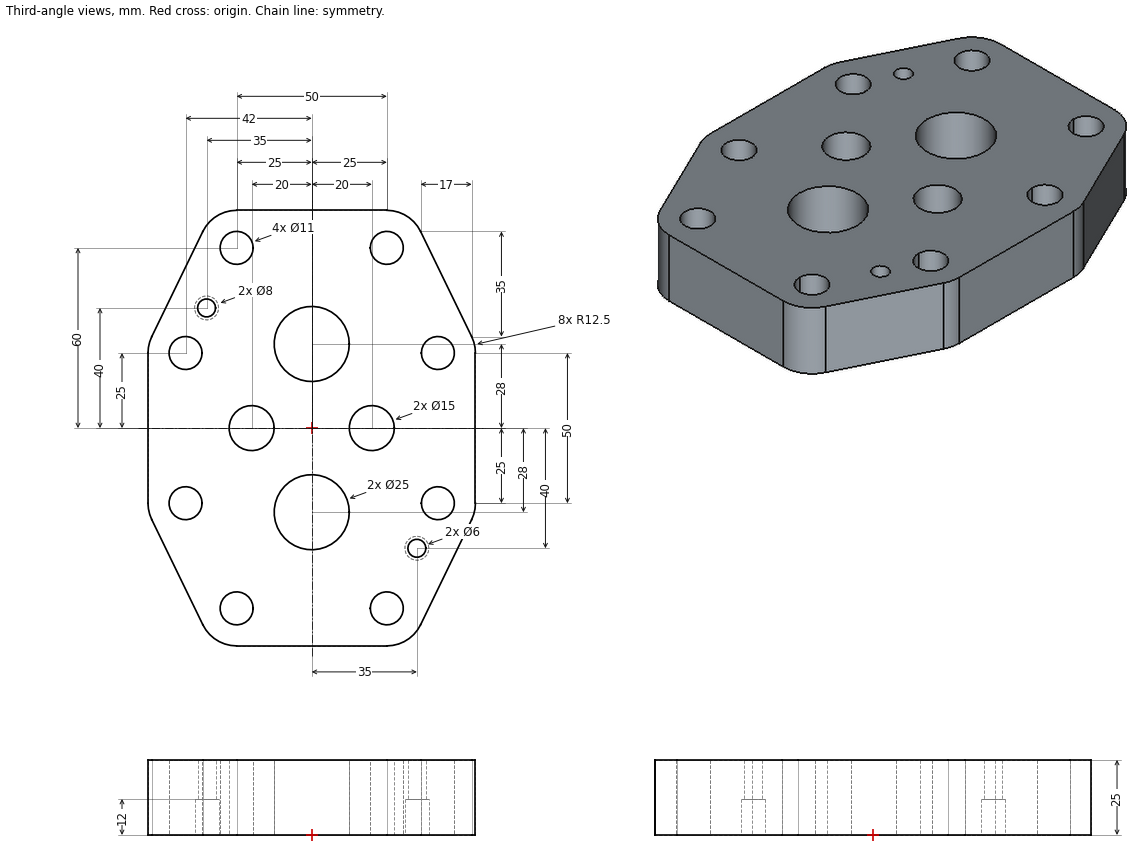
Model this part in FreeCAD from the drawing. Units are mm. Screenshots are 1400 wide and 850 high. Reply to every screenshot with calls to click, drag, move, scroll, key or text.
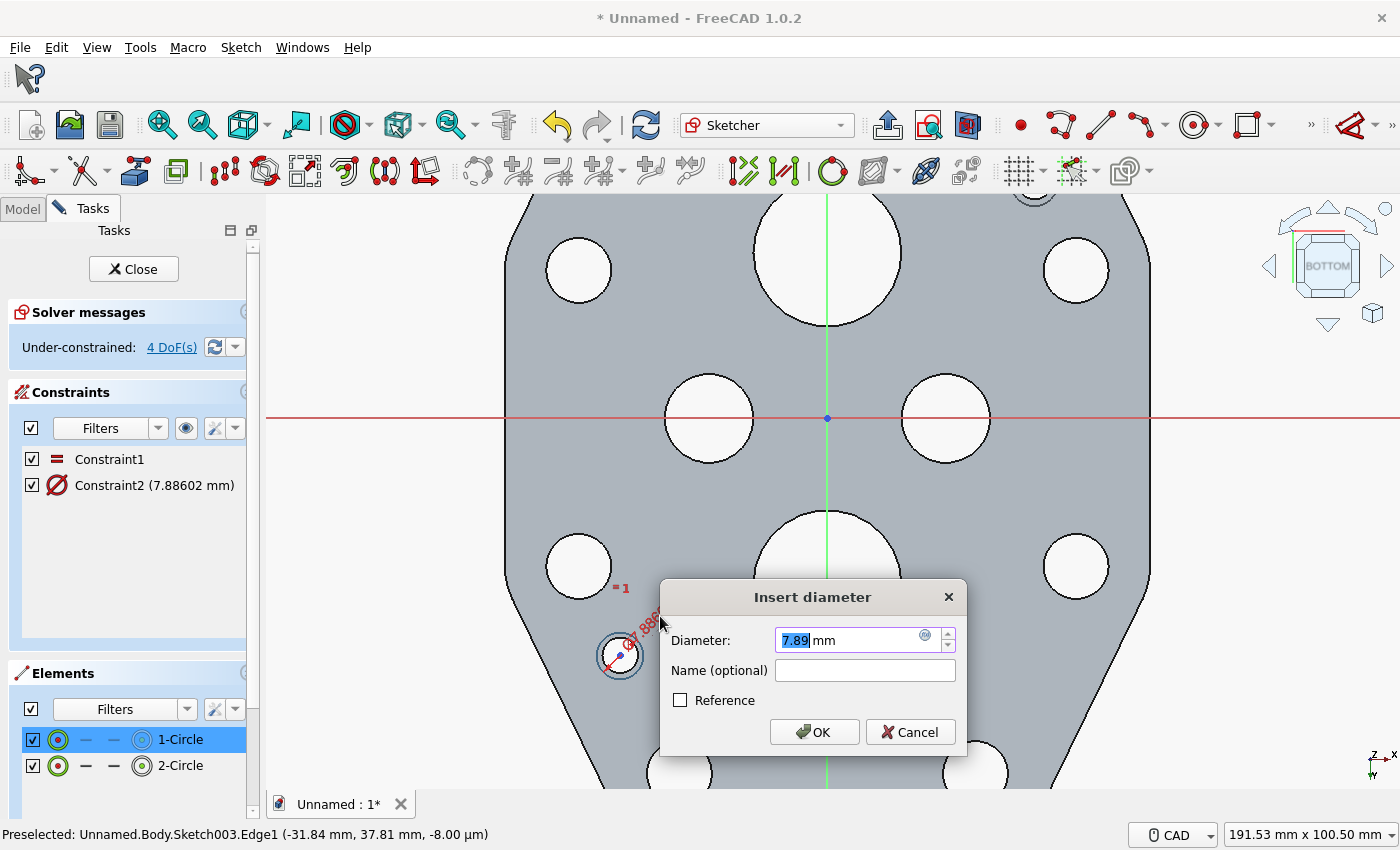
text(8)
key(Return)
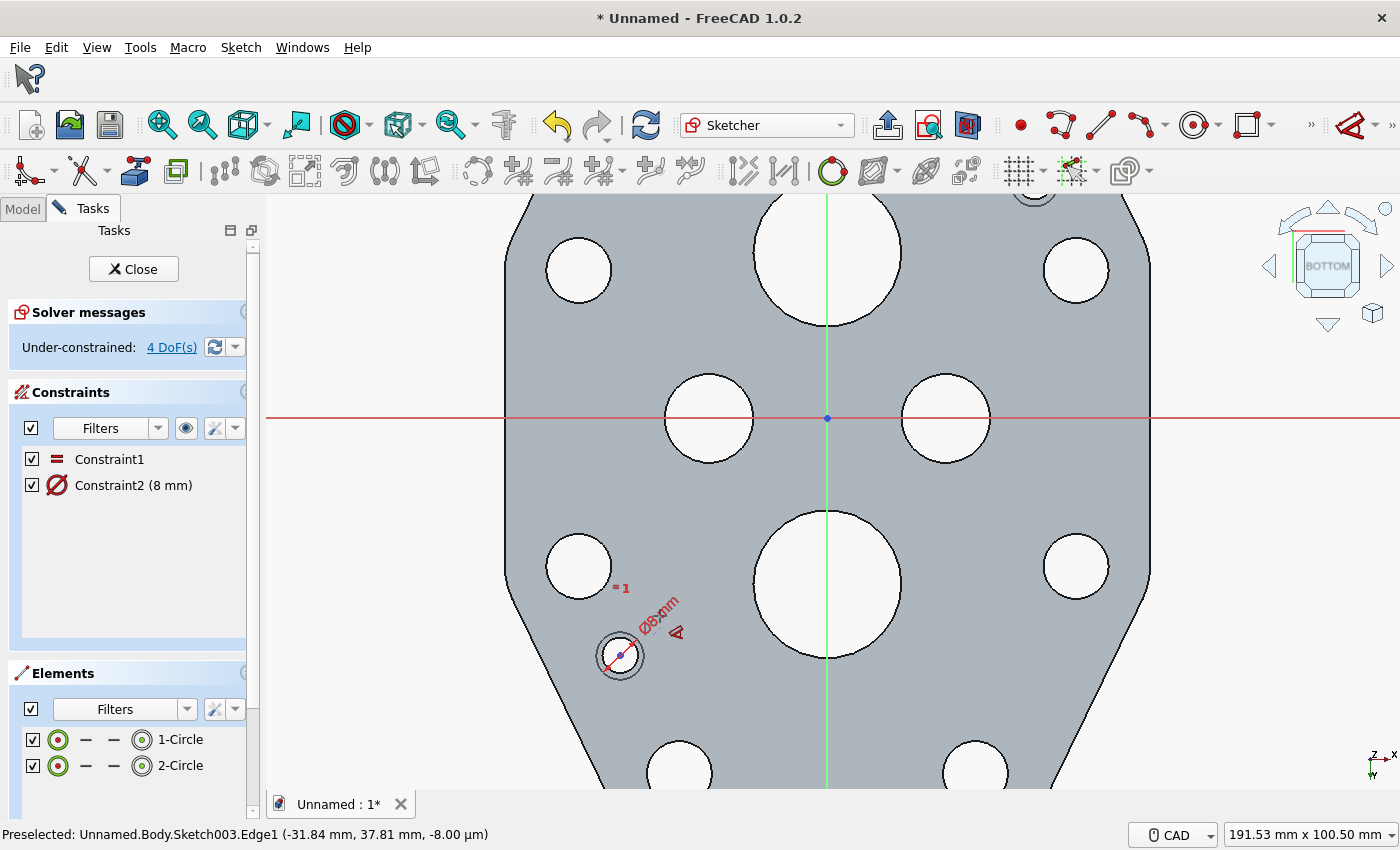
click(620, 656)
click(724, 690)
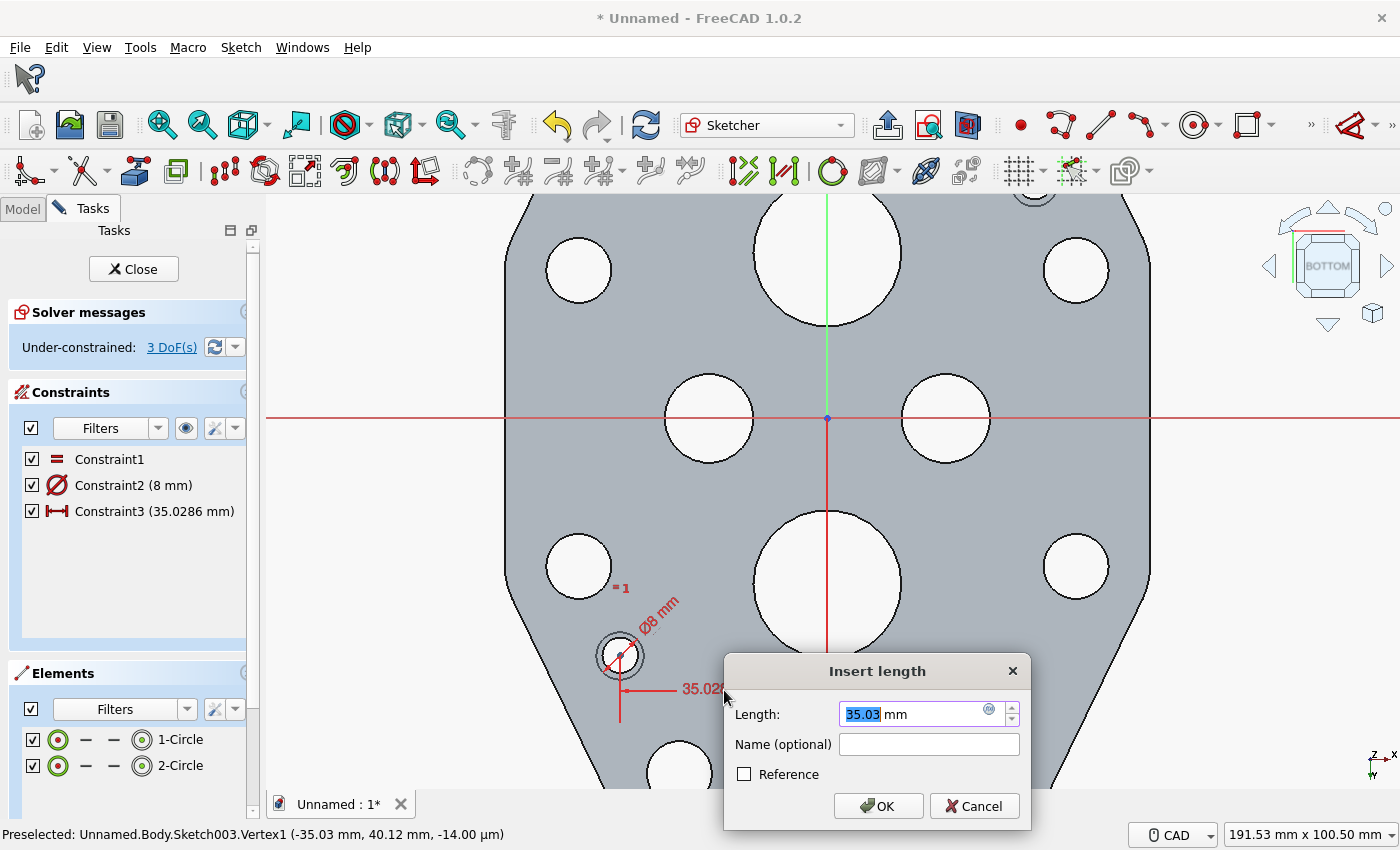
text(35)
key(Return)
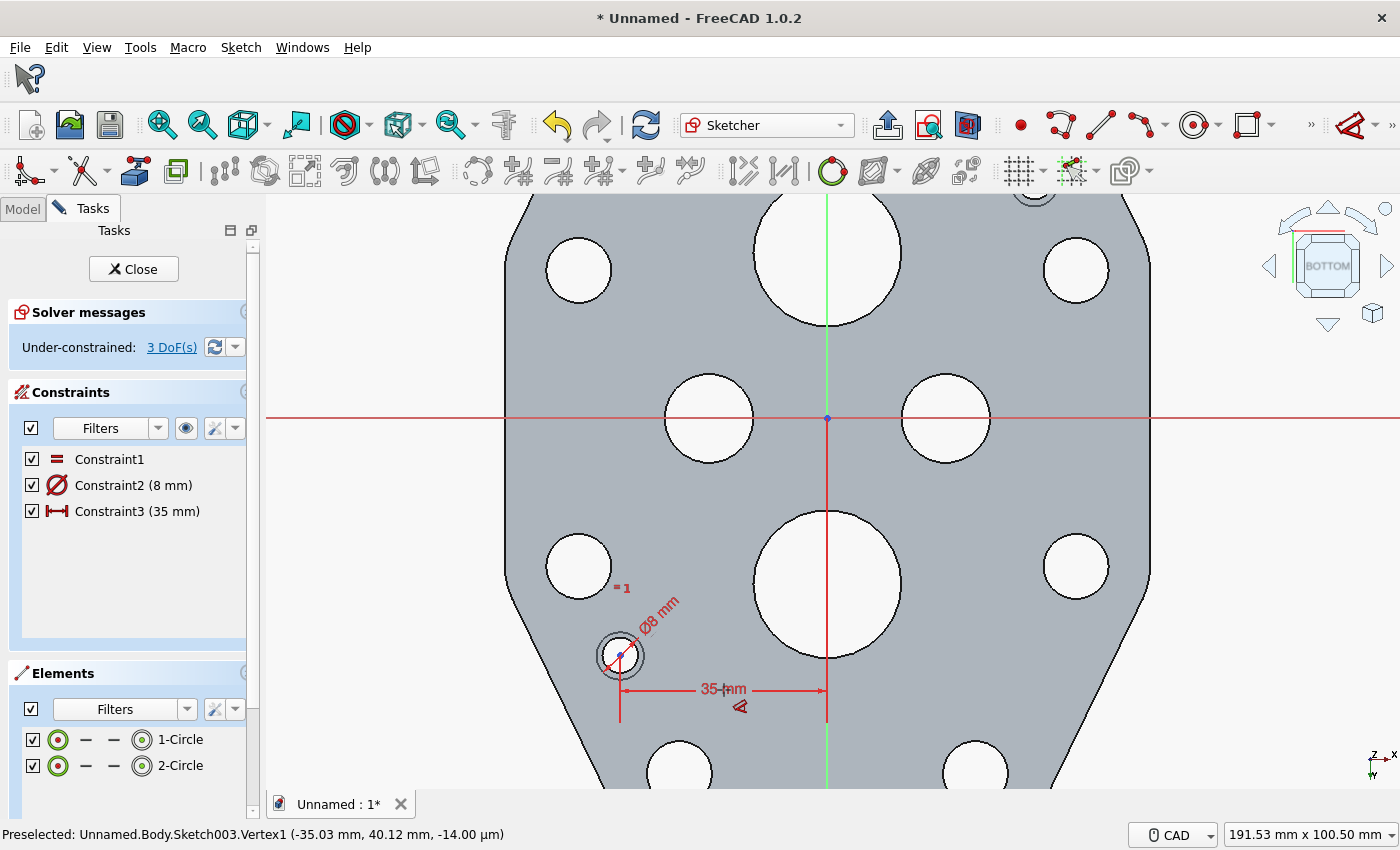
click(620, 656)
click(586, 537)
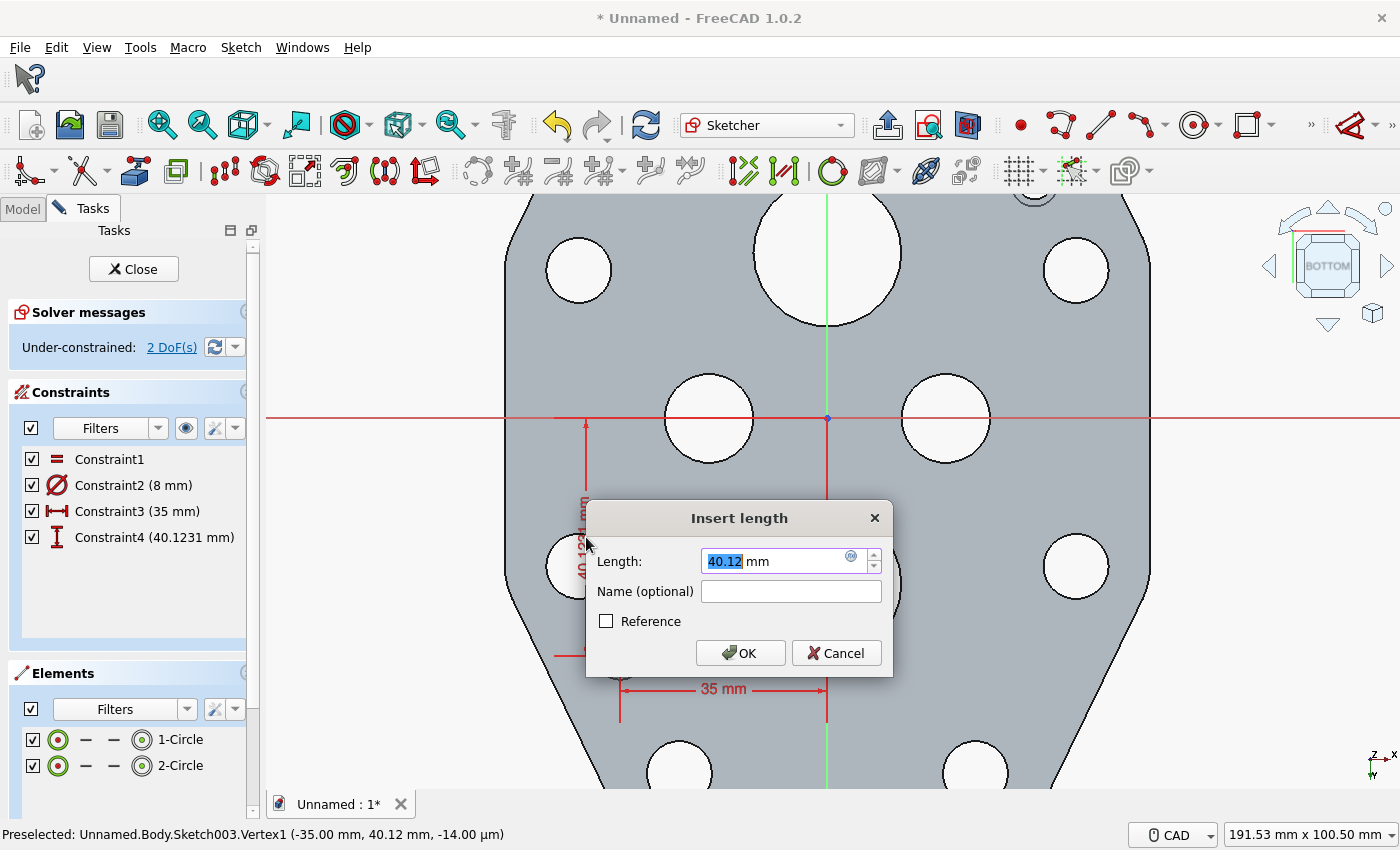
text(40)
key(Return)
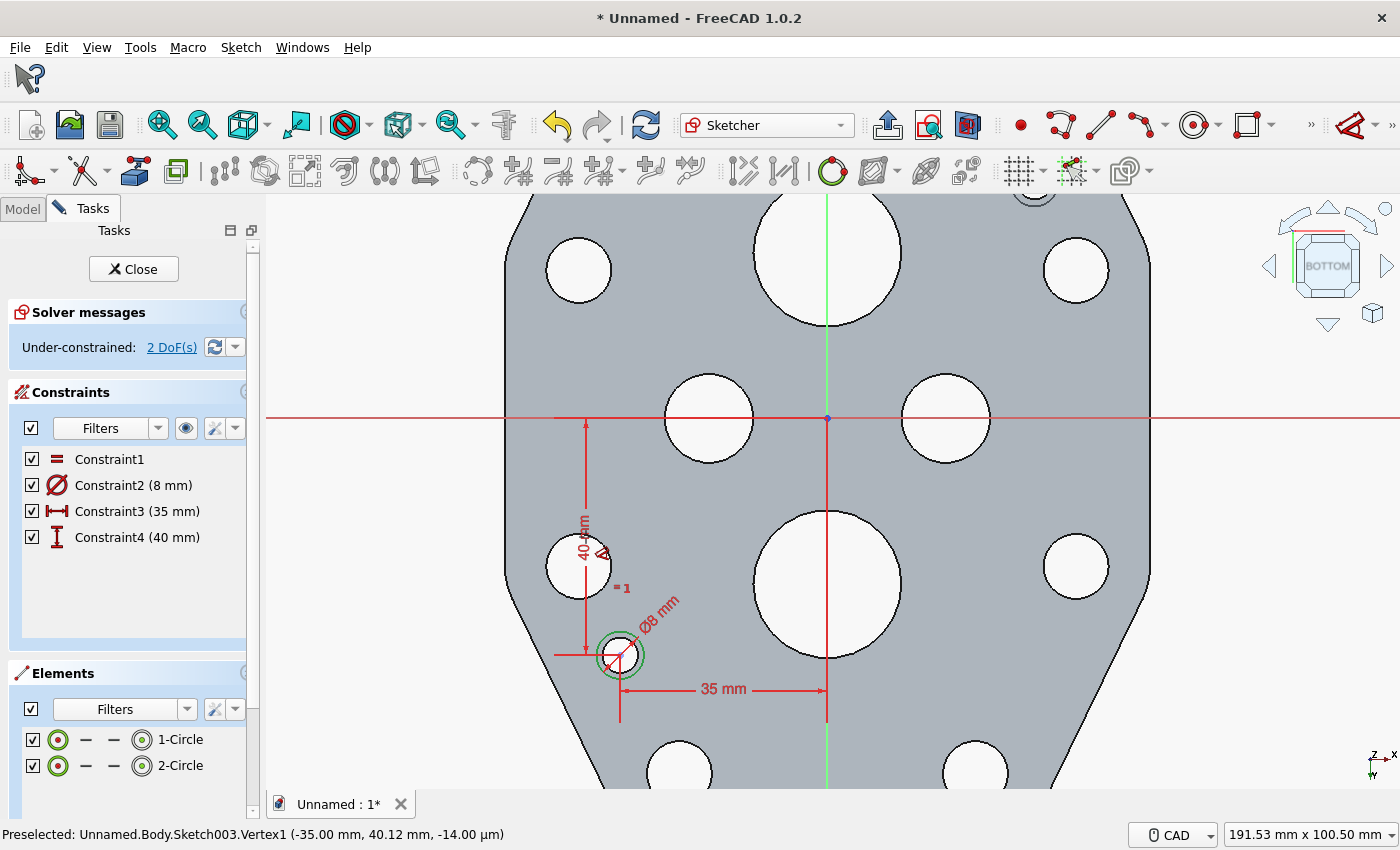
scroll(637, 640, down, 2)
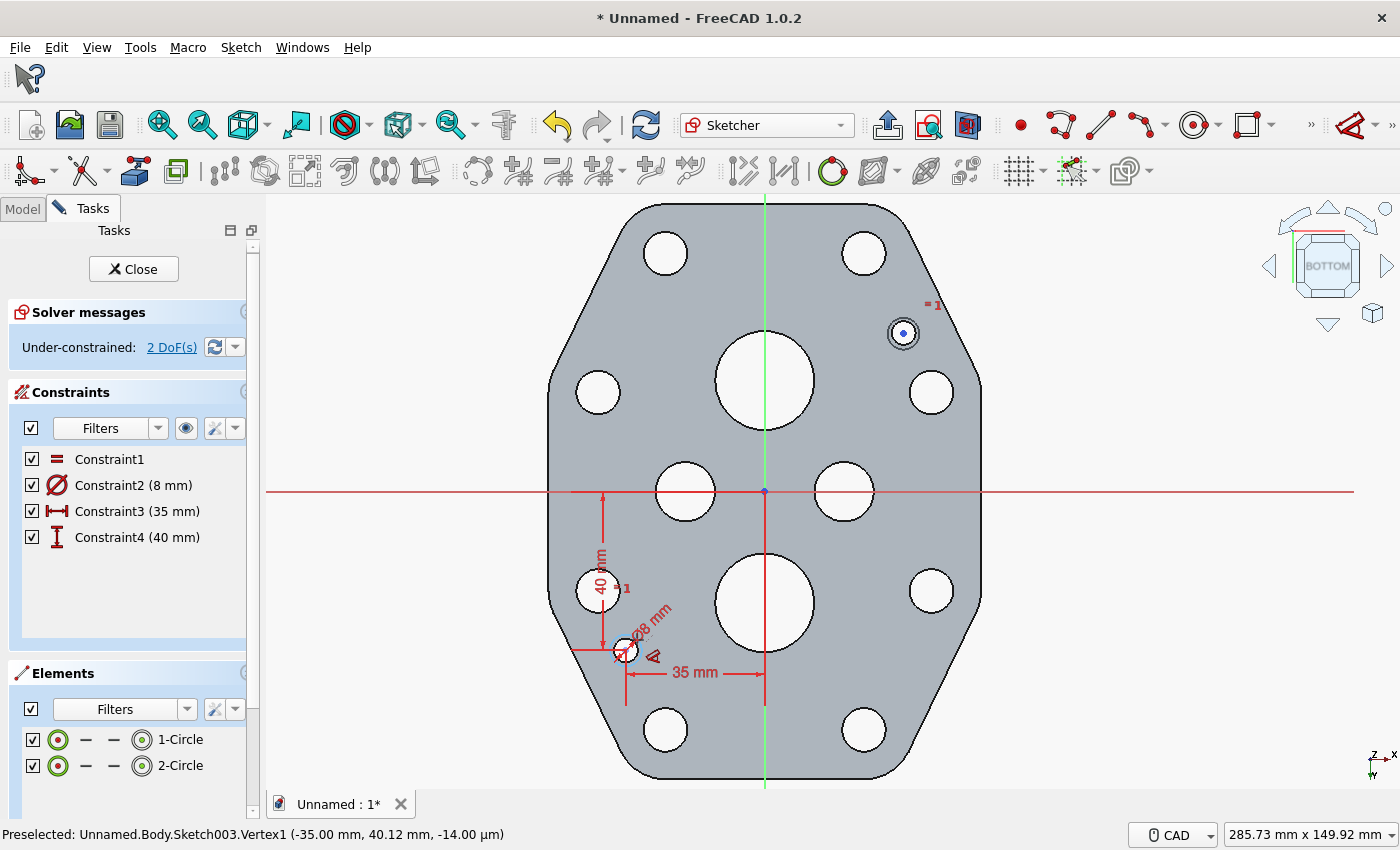
click(904, 334)
click(834, 300)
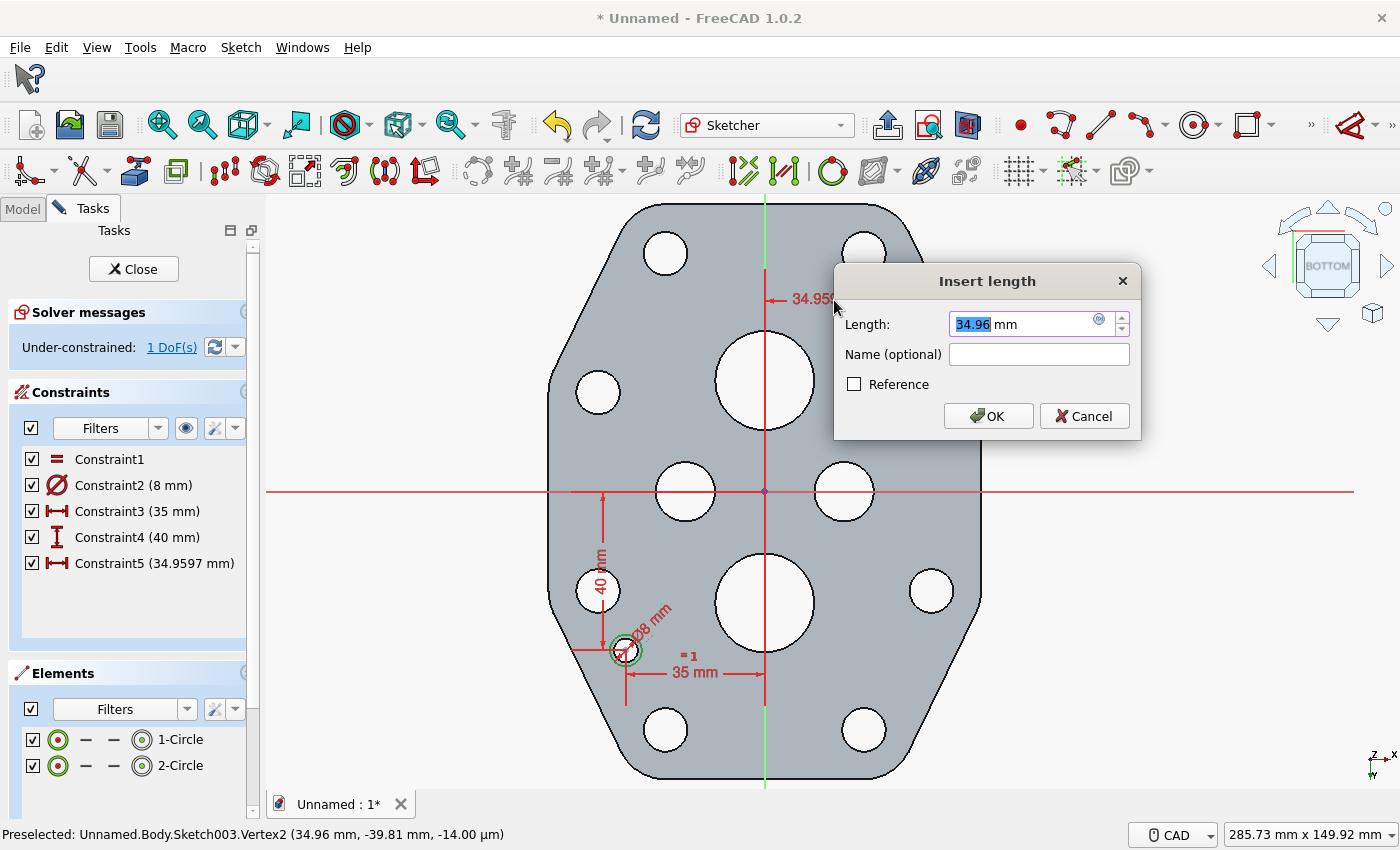
text(35)
key(Return)